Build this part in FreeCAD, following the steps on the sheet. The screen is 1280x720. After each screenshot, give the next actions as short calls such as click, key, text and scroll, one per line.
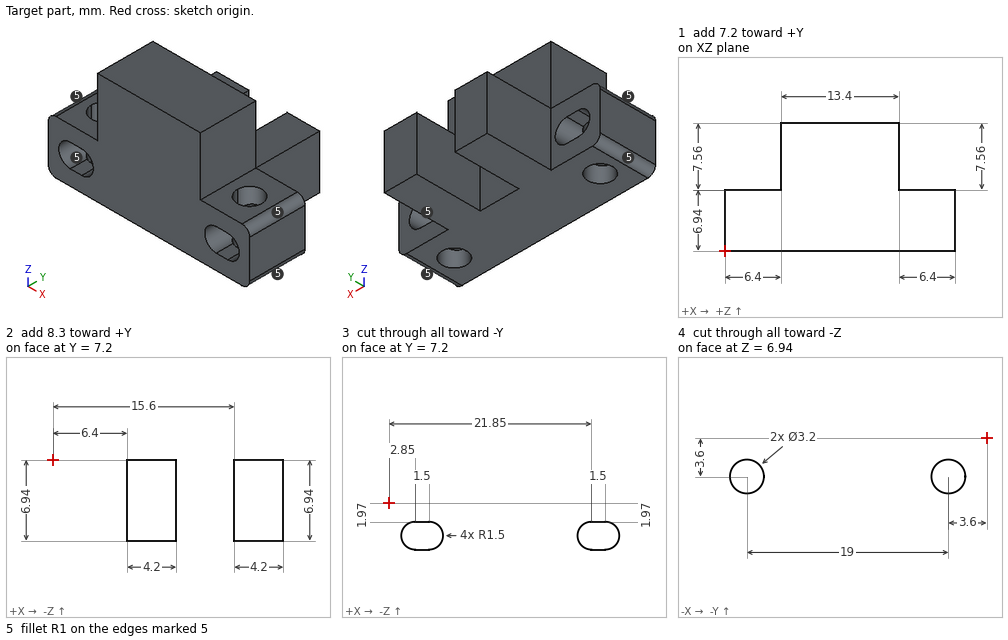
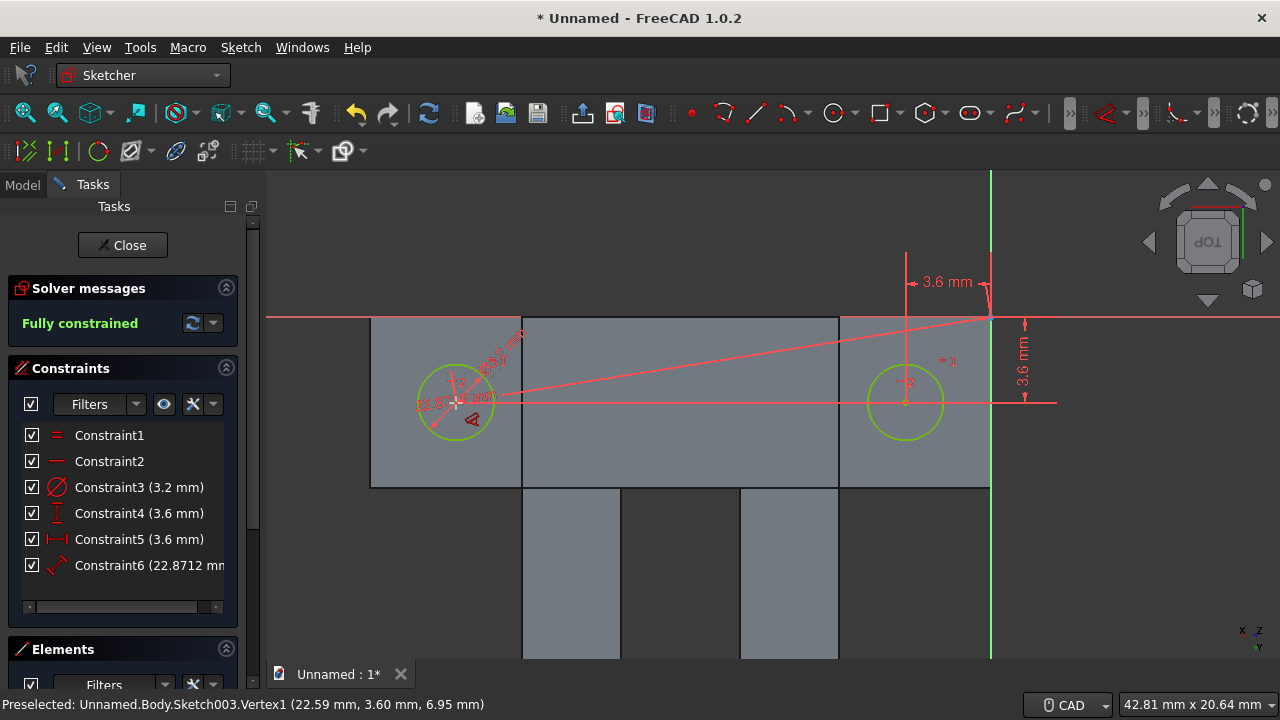
click(906, 403)
click(681, 437)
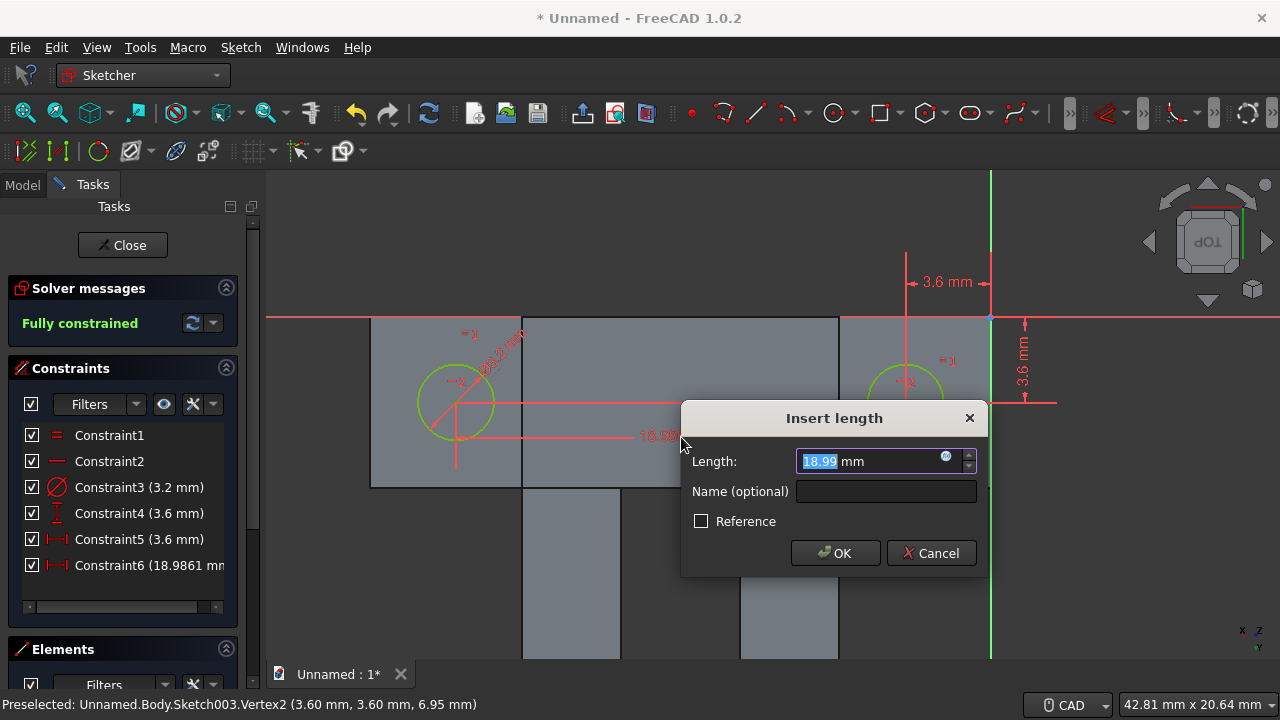
text(19)
key(Return)
key(Escape)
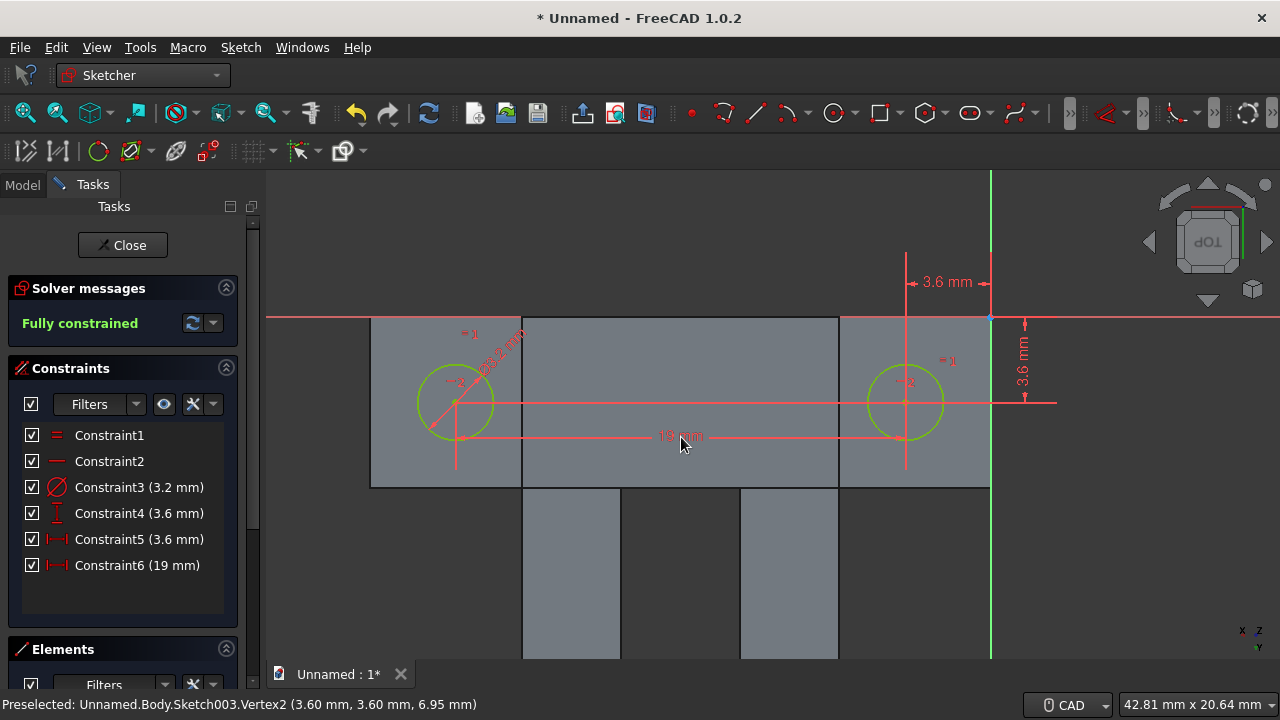
click(123, 245)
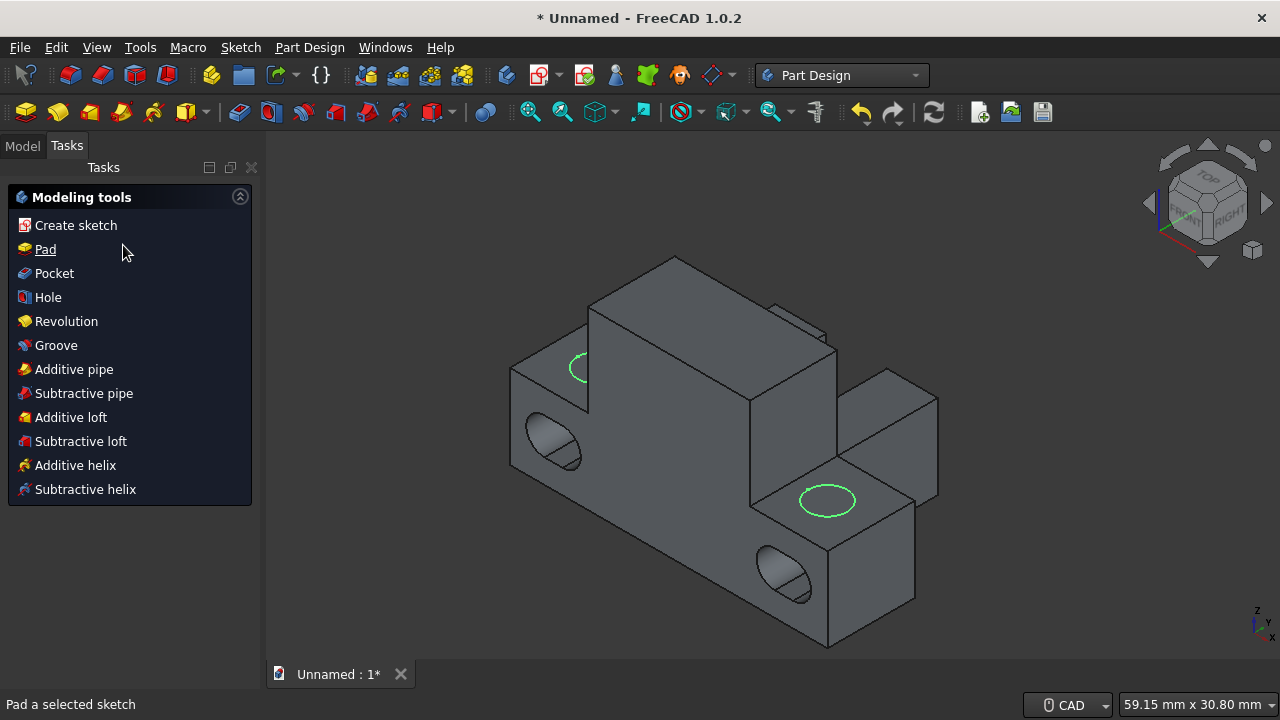
click(240, 112)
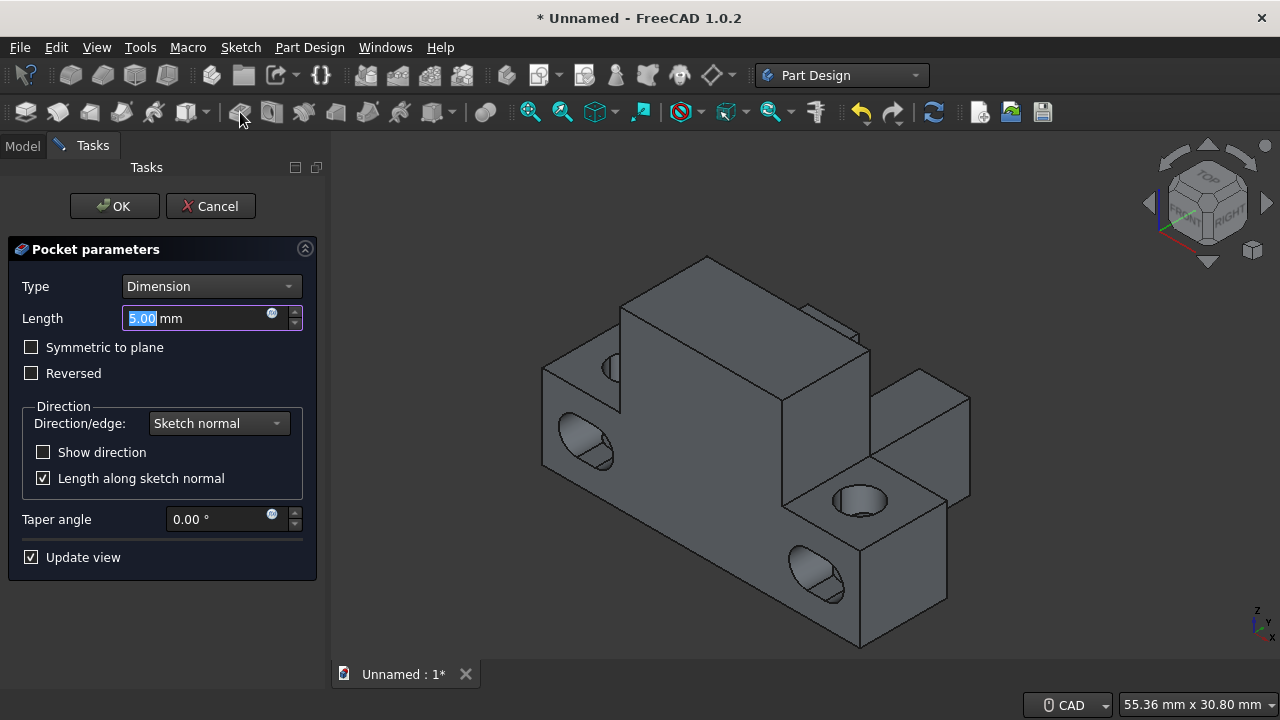
click(212, 286)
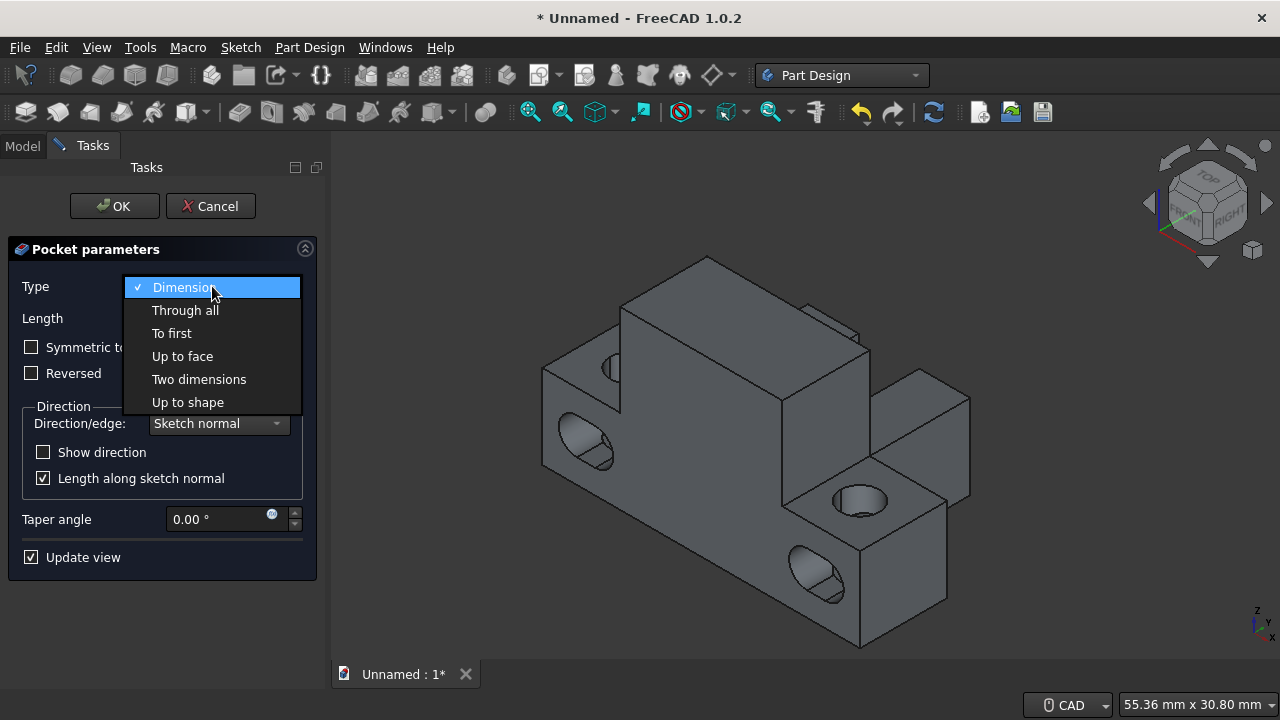
click(212, 310)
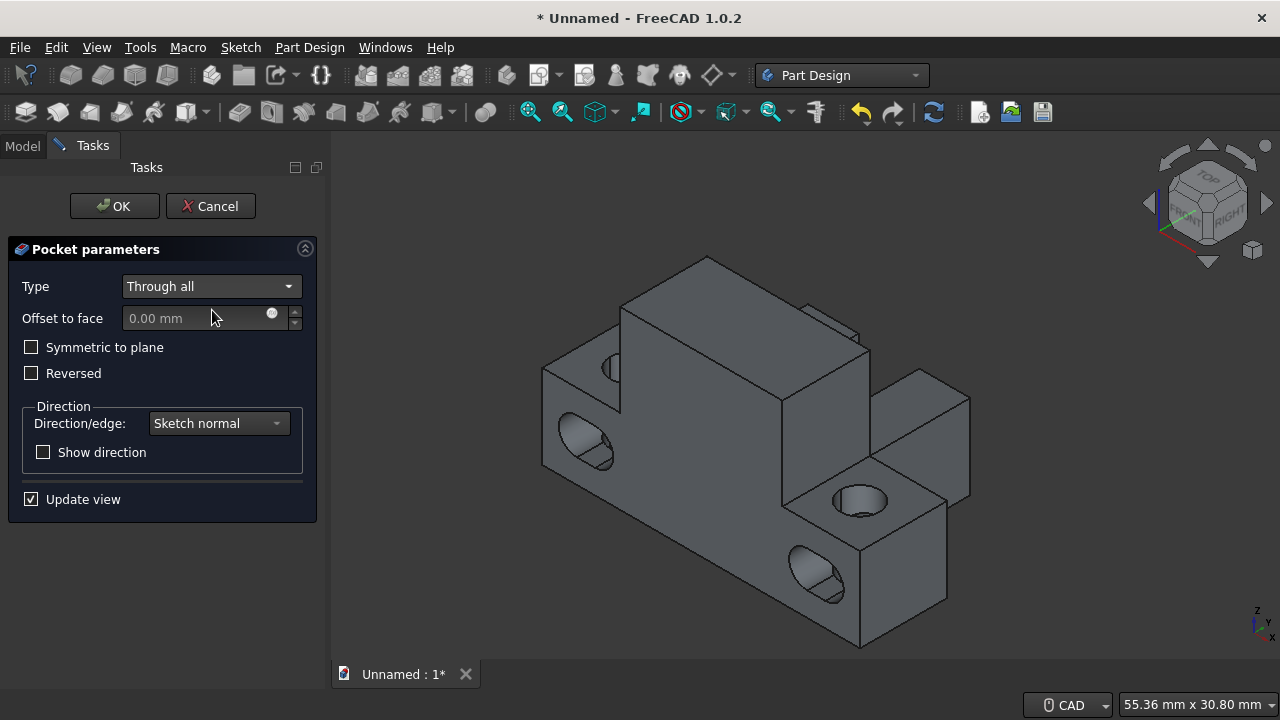
click(115, 206)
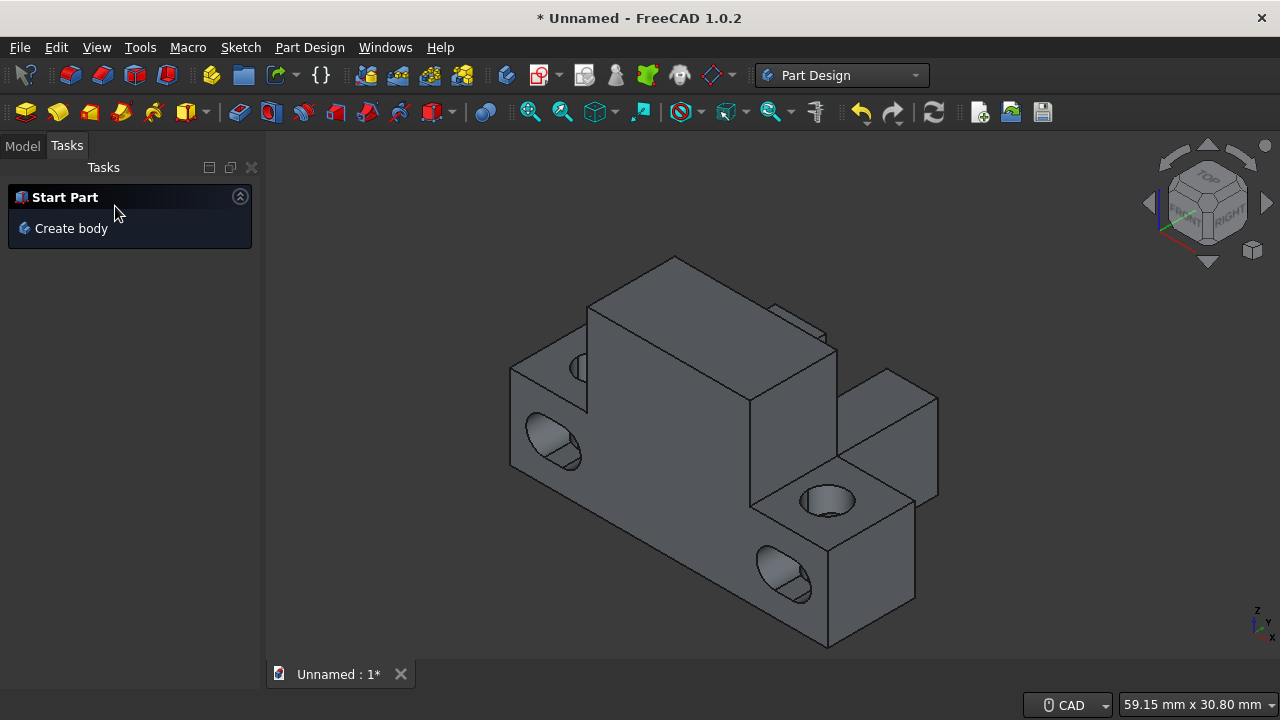
click(871, 525)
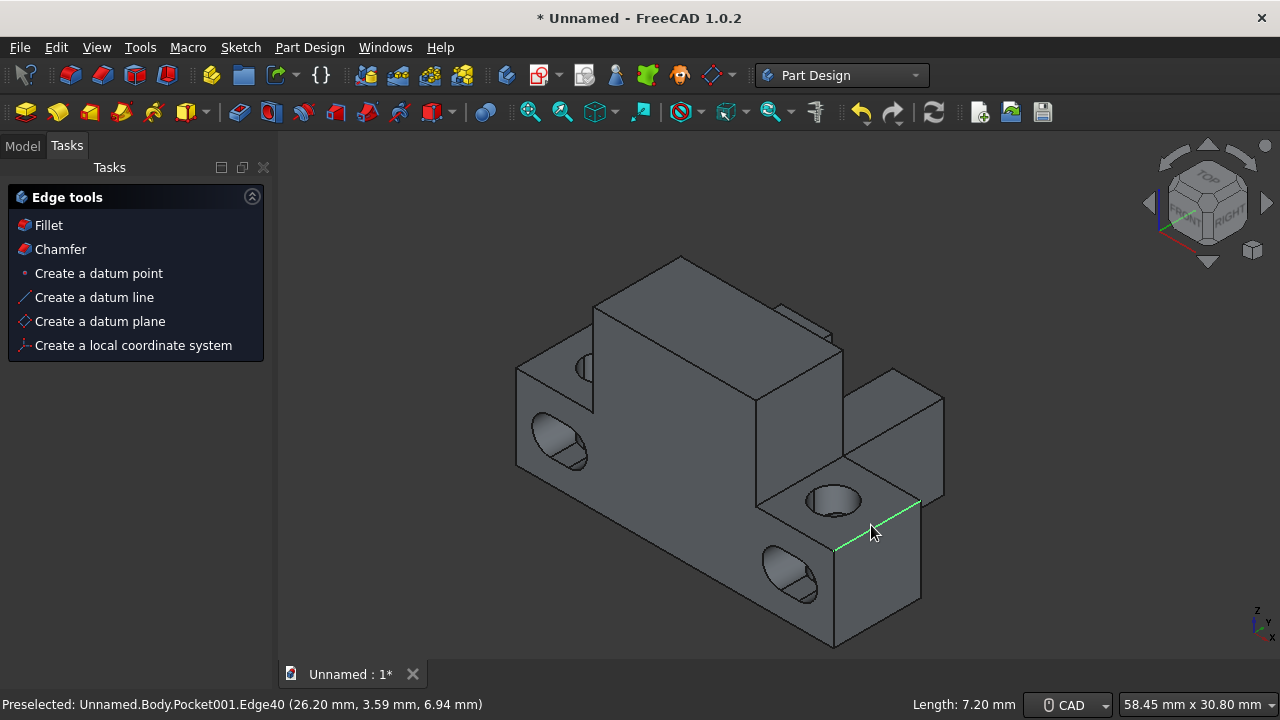
key(2)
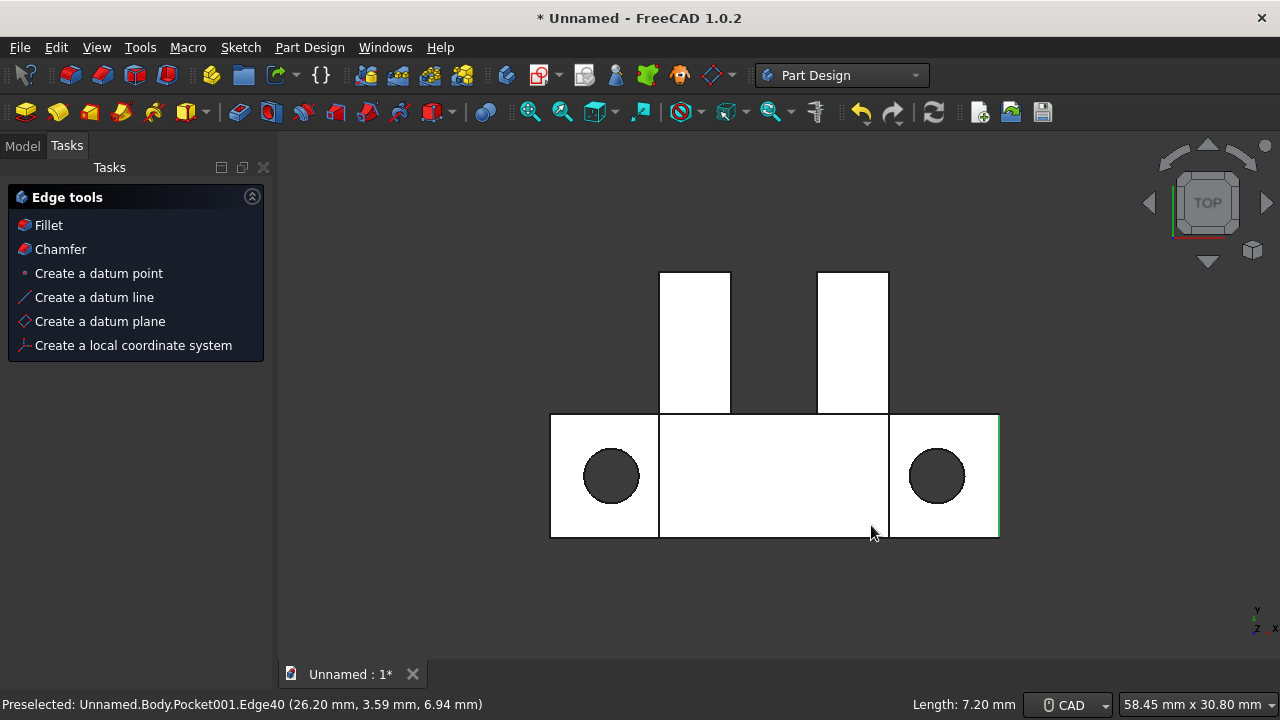
click(550, 475, ctrl)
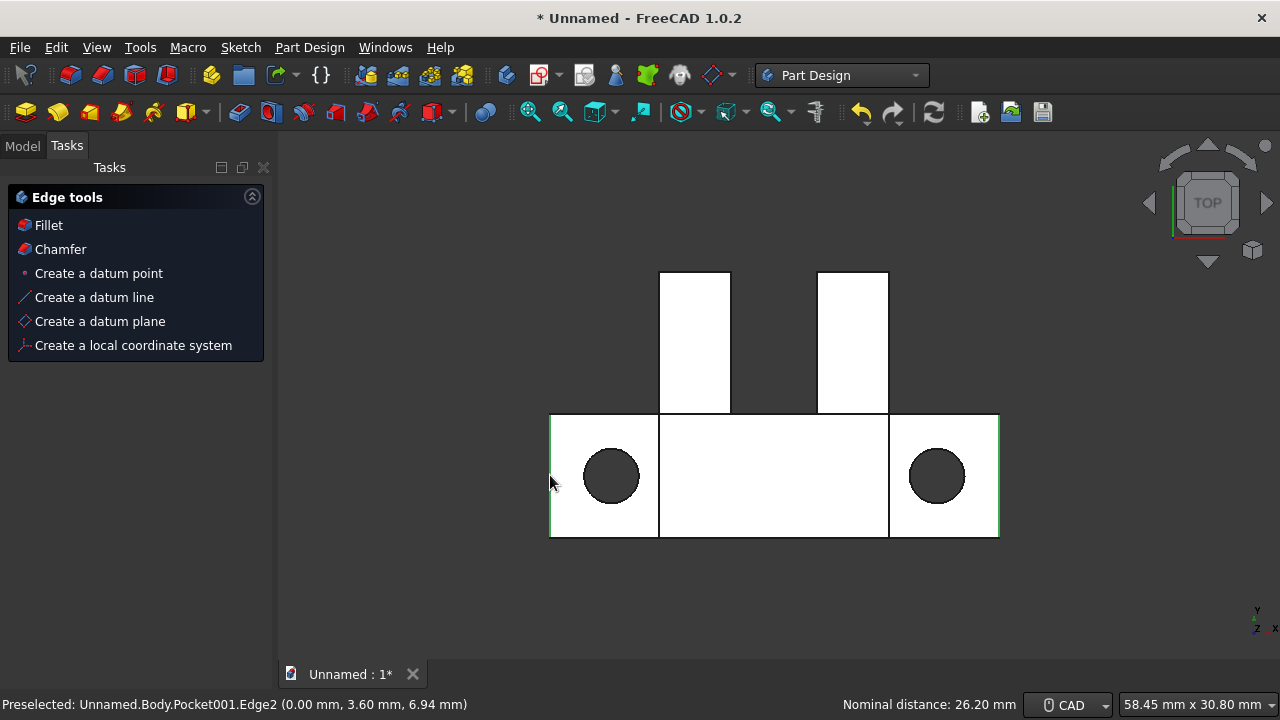
key(0)